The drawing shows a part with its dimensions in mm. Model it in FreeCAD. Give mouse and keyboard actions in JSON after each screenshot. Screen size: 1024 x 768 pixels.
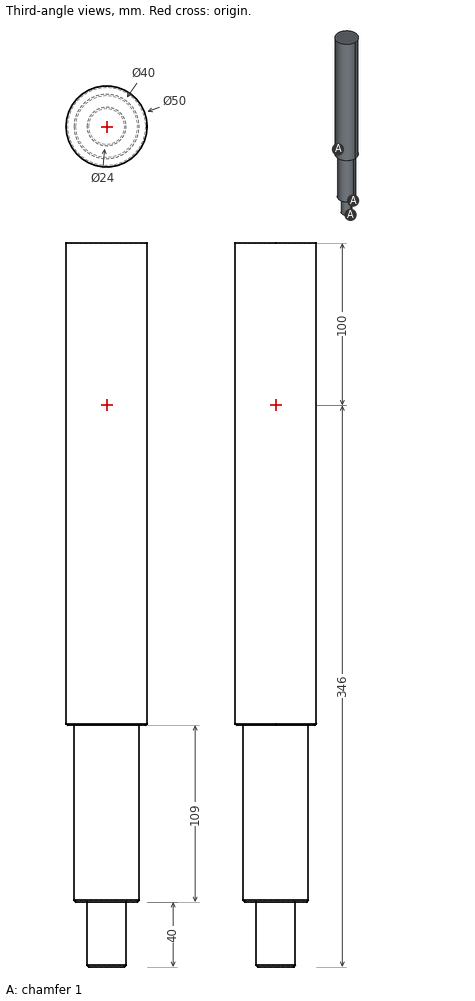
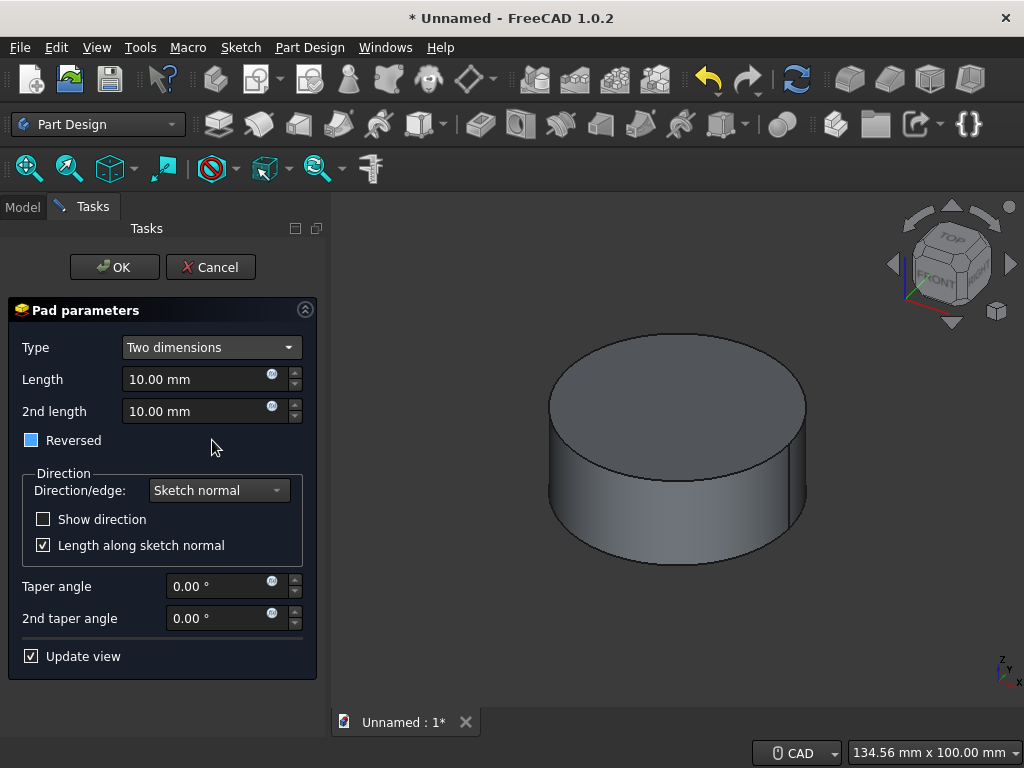
{"action": "triple_click", "coordinate": [204, 379]}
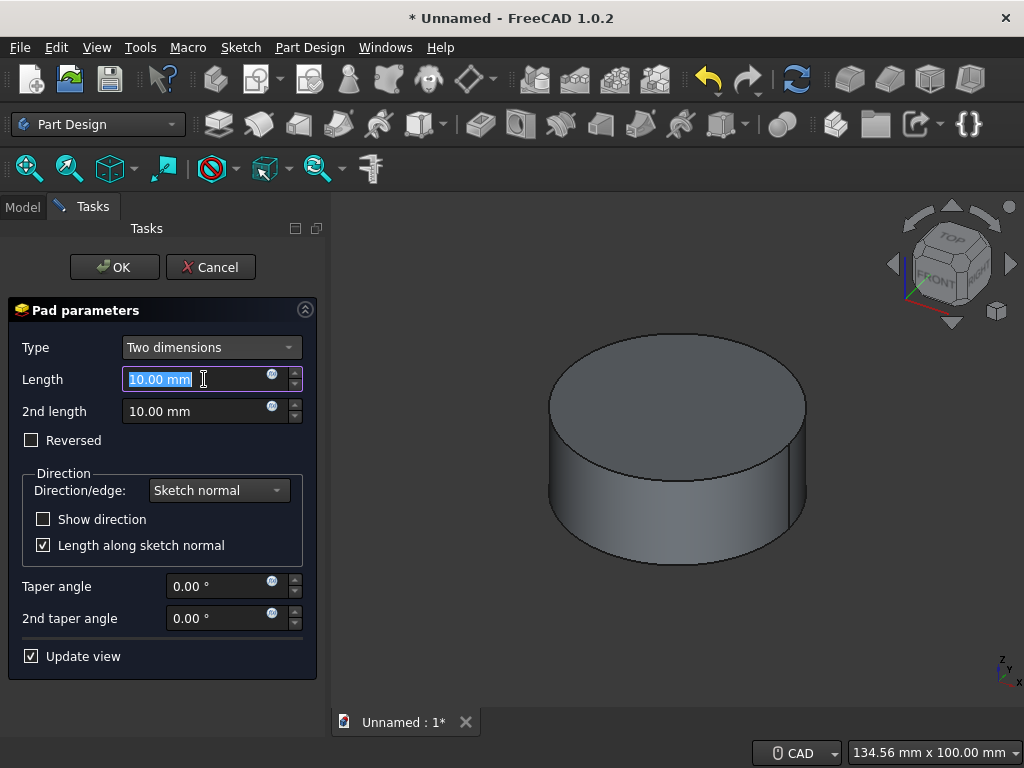
{"action": "type", "text": "100"}
{"action": "key", "text": "Tab"}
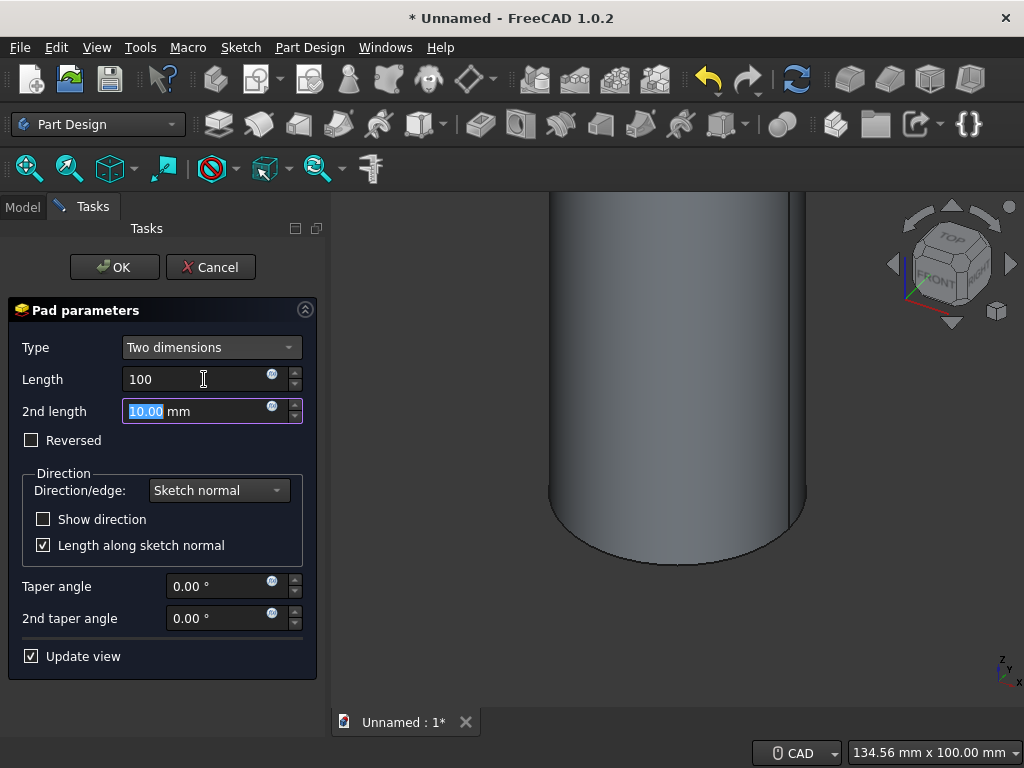
{"action": "type", "text": "346"}
{"action": "key", "text": "Tab"}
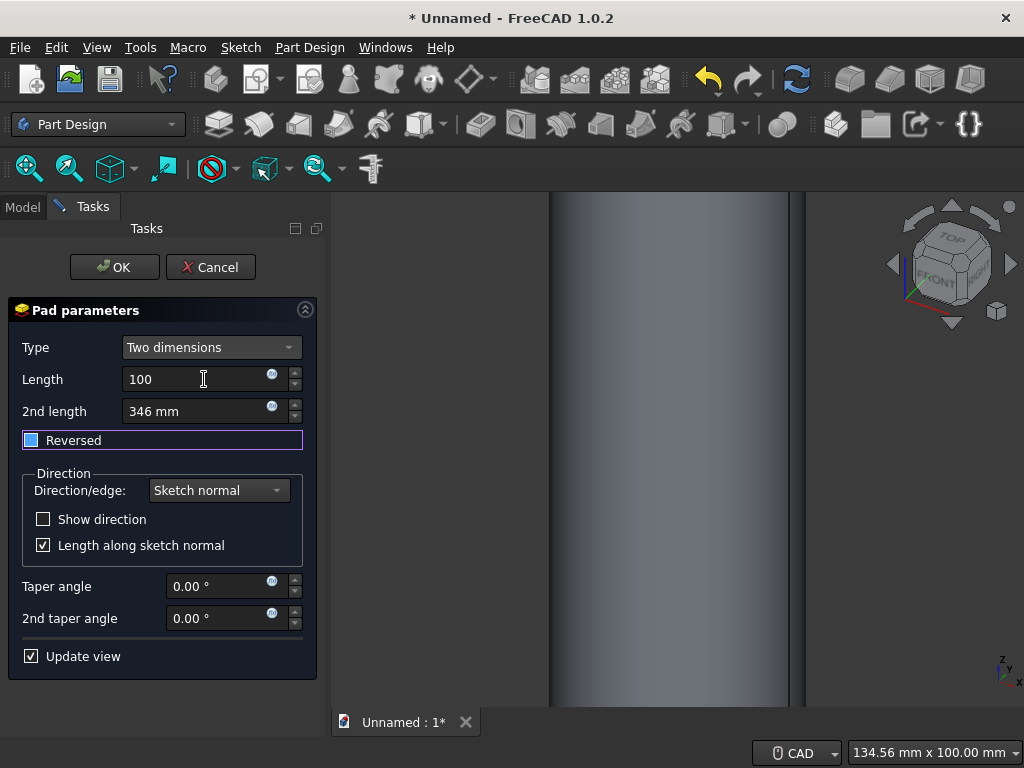
{"action": "left_click", "coordinate": [115, 267]}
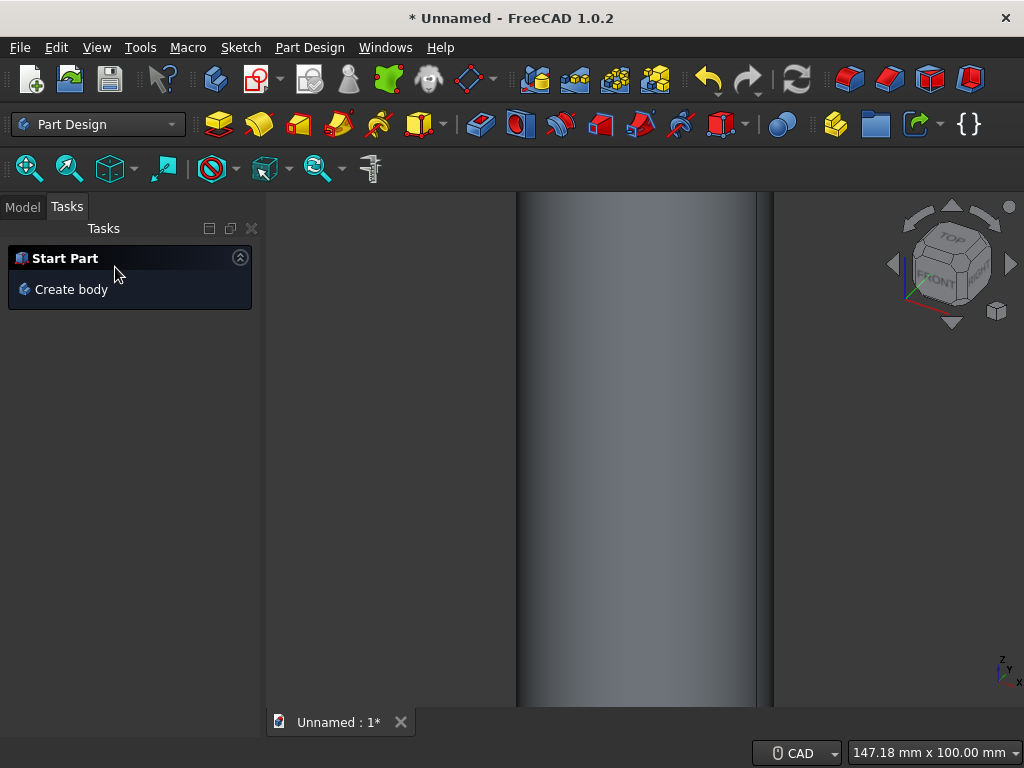
{"action": "left_click", "coordinate": [30, 170]}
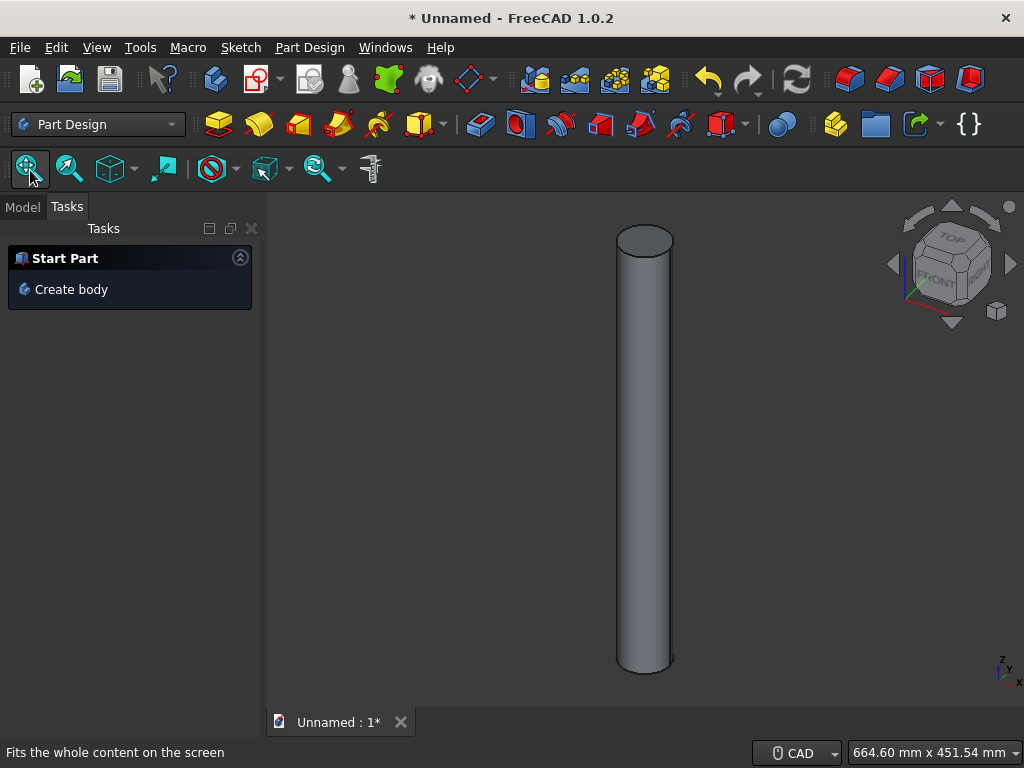
{"action": "left_click", "coordinate": [23, 206]}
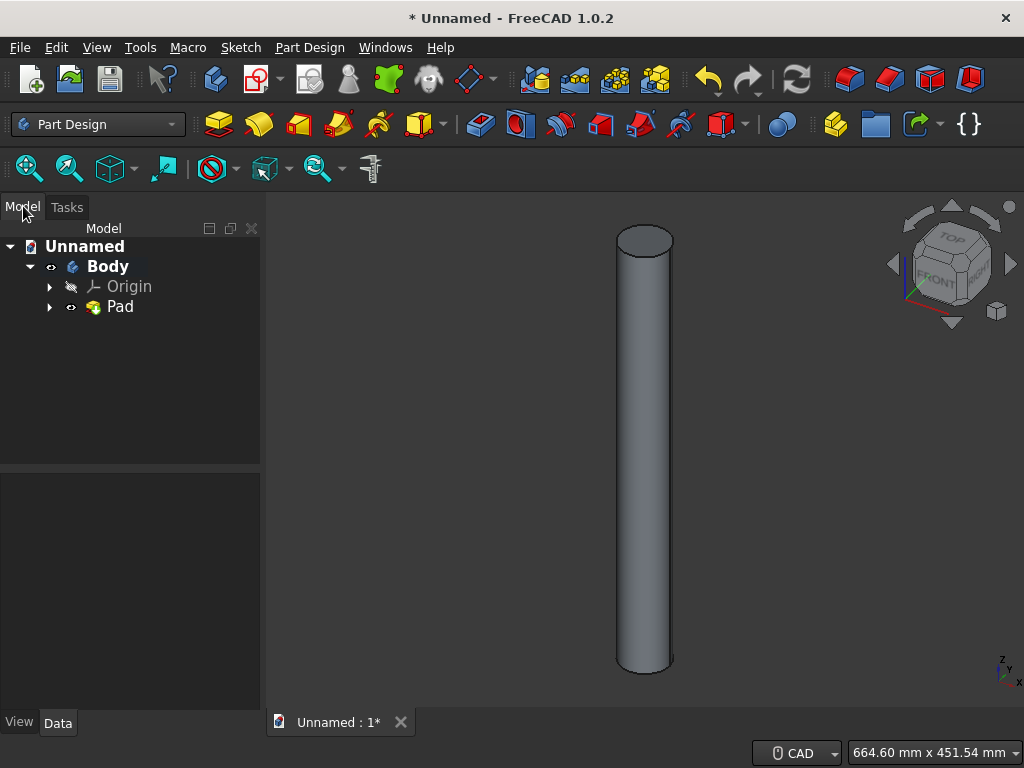
{"action": "left_click", "coordinate": [50, 287]}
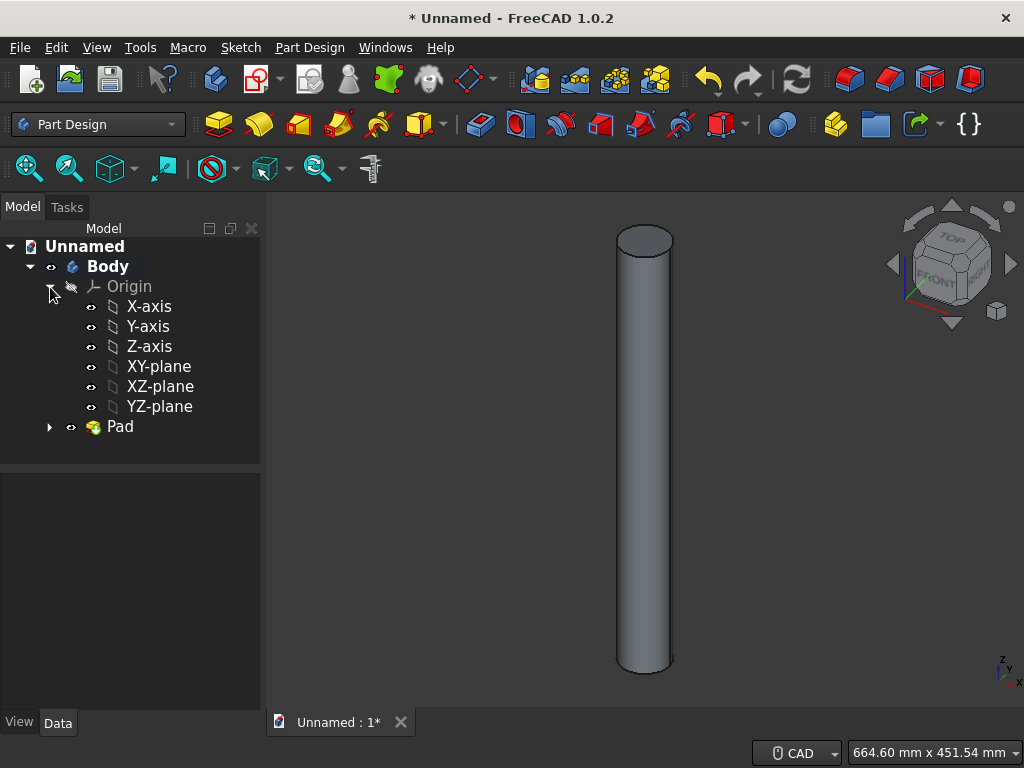
{"action": "left_click", "coordinate": [136, 367]}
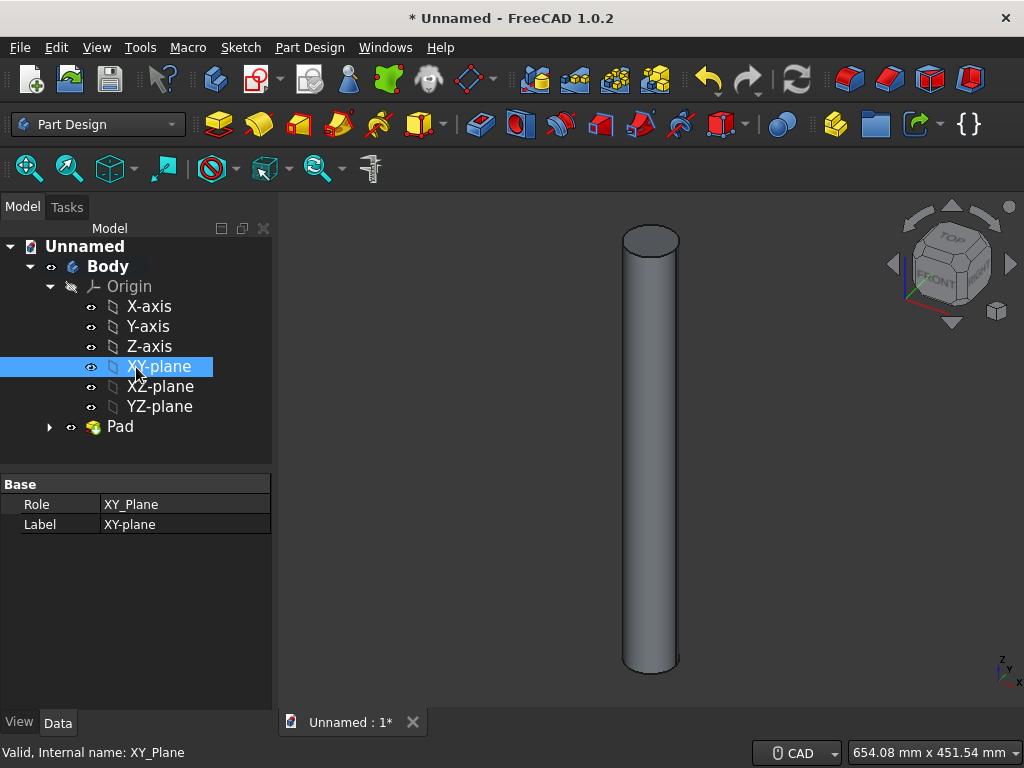
{"action": "left_click", "coordinate": [470, 80]}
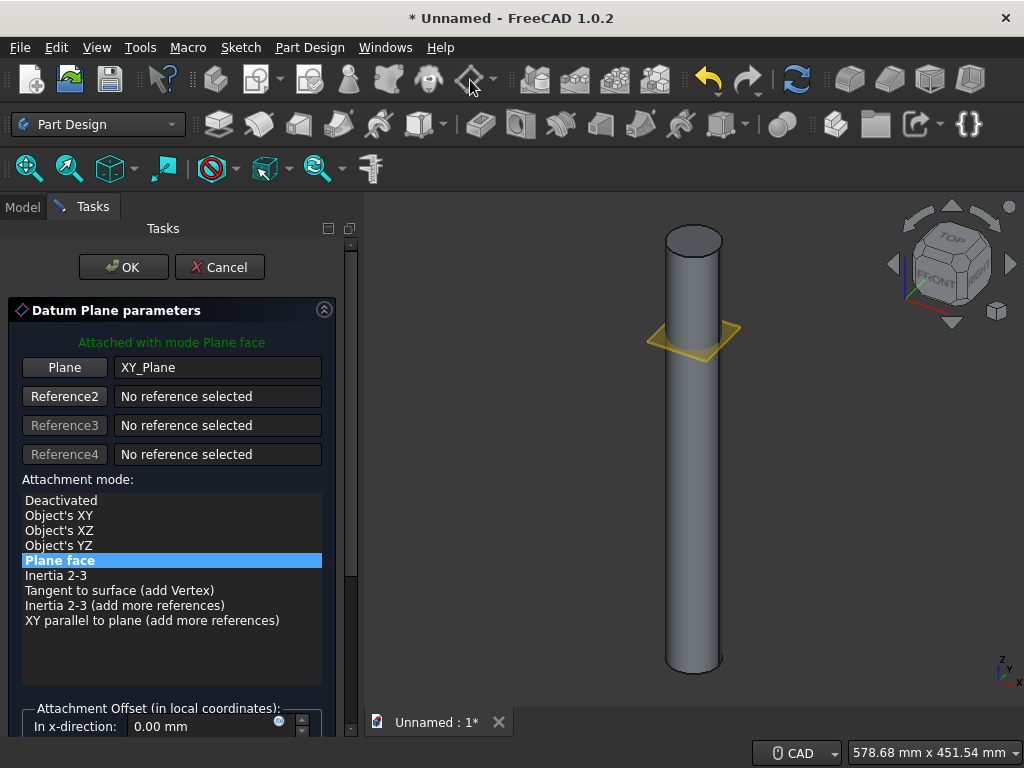
{"action": "scroll", "coordinate": [351, 487], "scroll_direction": "down", "scroll_amount": 3}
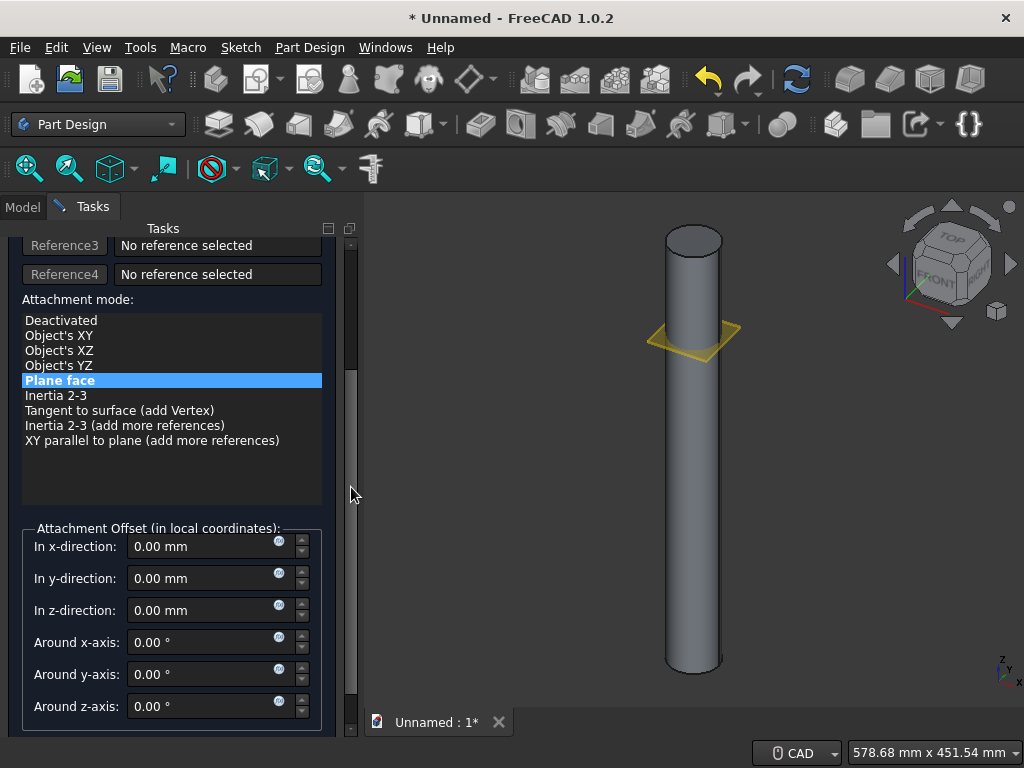
{"action": "triple_click", "coordinate": [210, 610]}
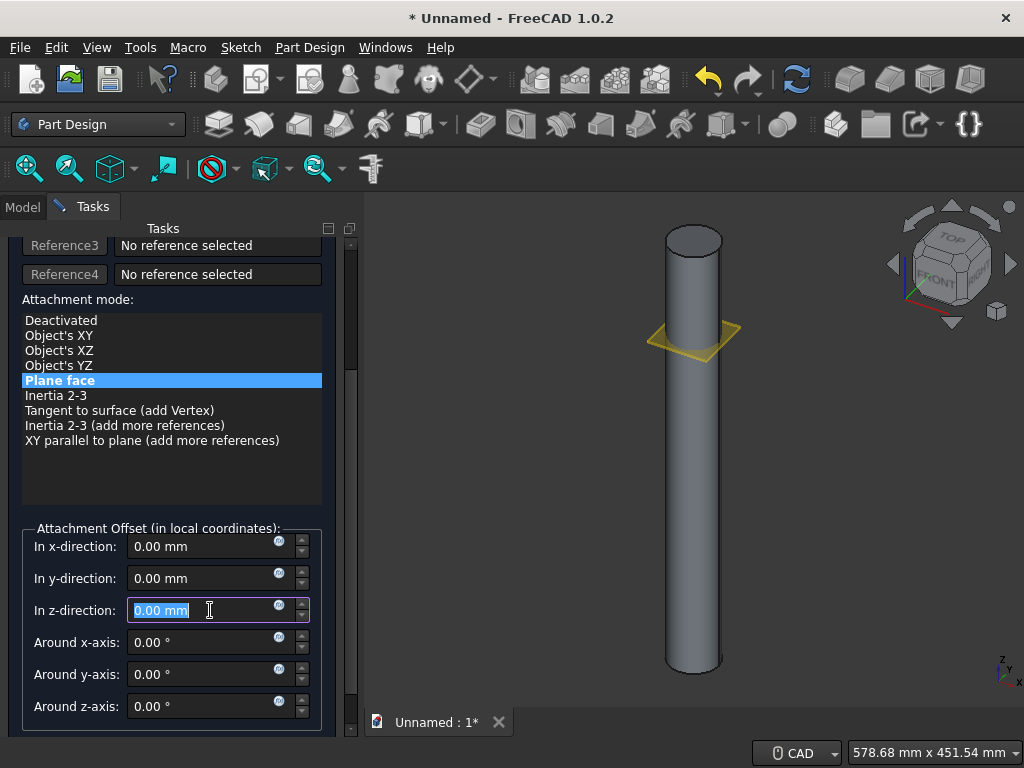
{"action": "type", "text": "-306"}
{"action": "key", "text": "Tab"}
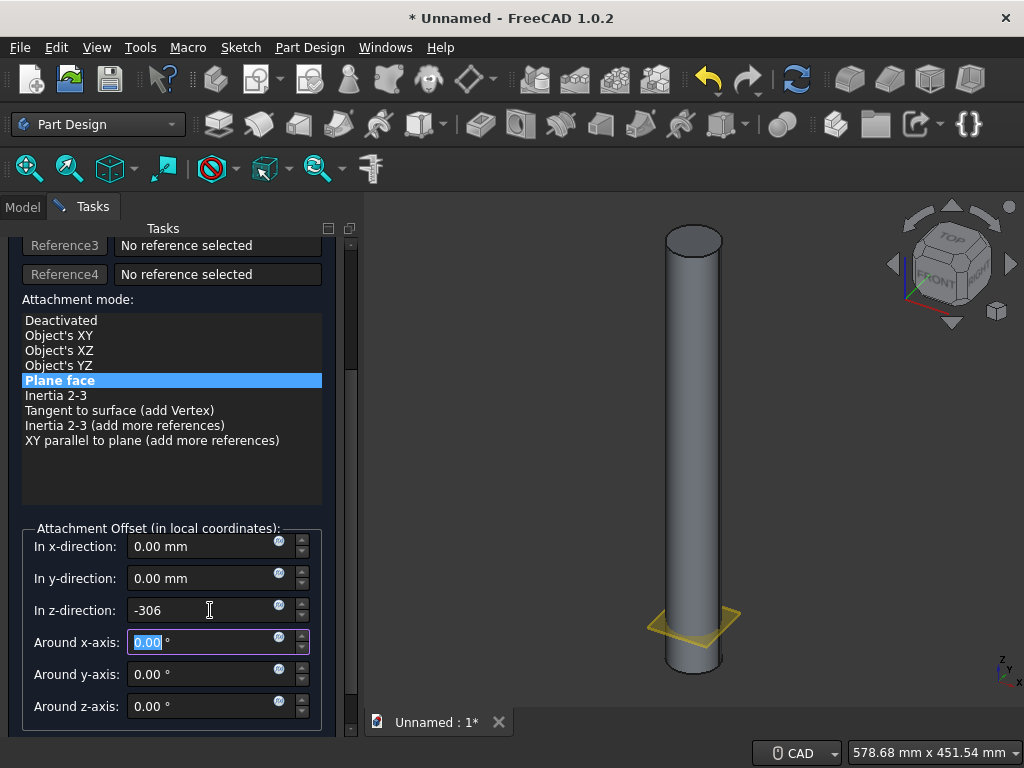
{"action": "scroll", "coordinate": [351, 487], "scroll_direction": "up", "scroll_amount": 4}